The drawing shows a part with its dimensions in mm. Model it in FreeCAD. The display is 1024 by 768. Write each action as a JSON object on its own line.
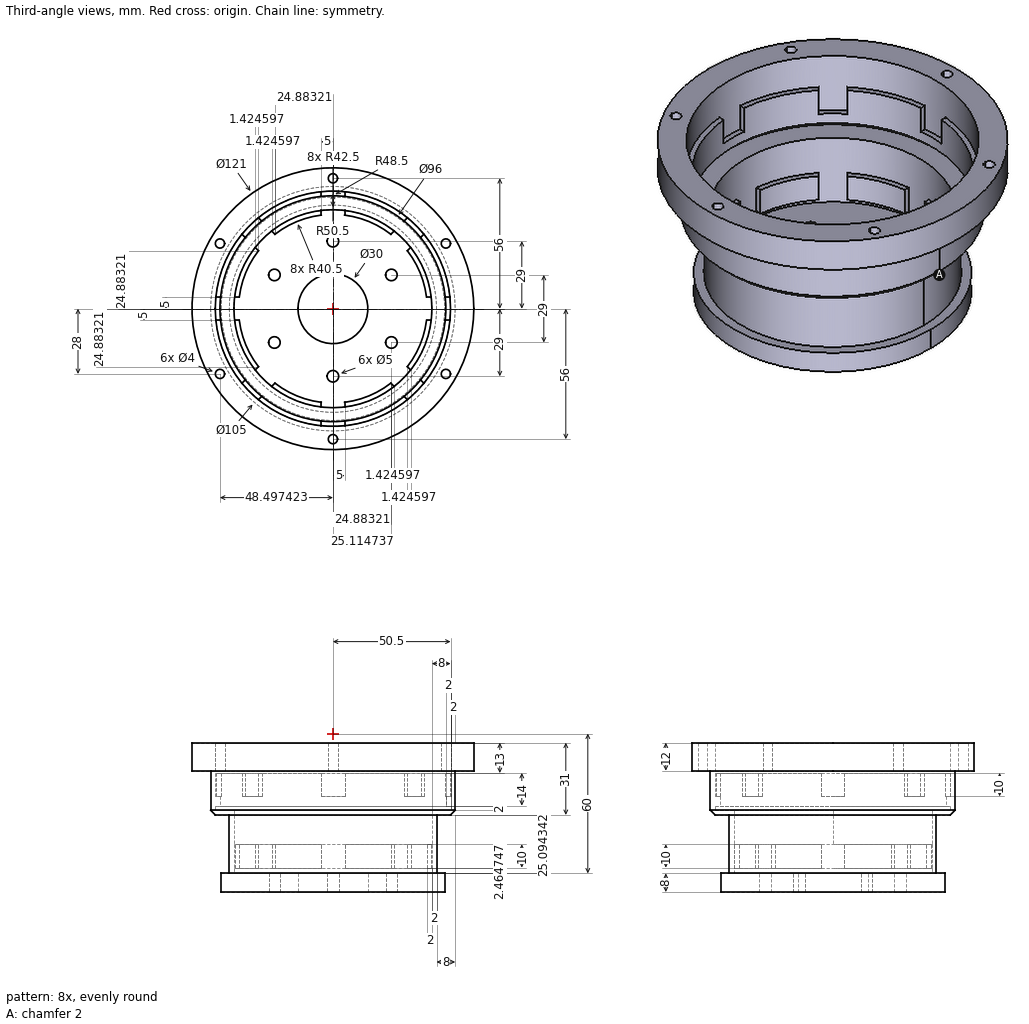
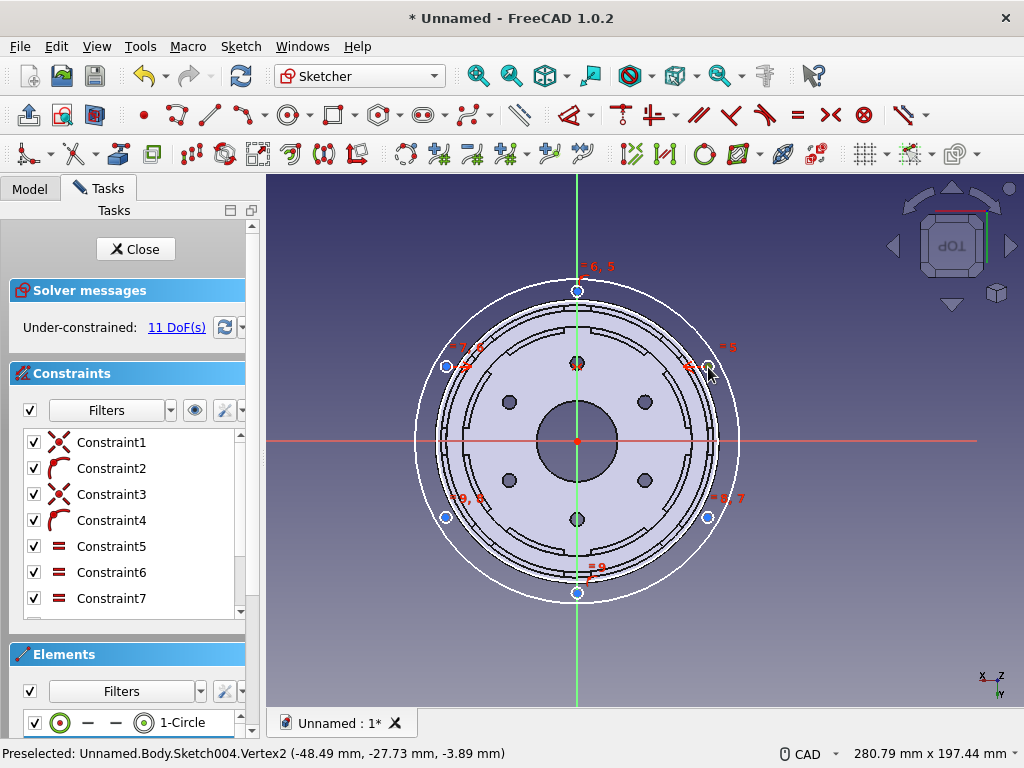
{"action": "left_click", "coordinate": [708, 518]}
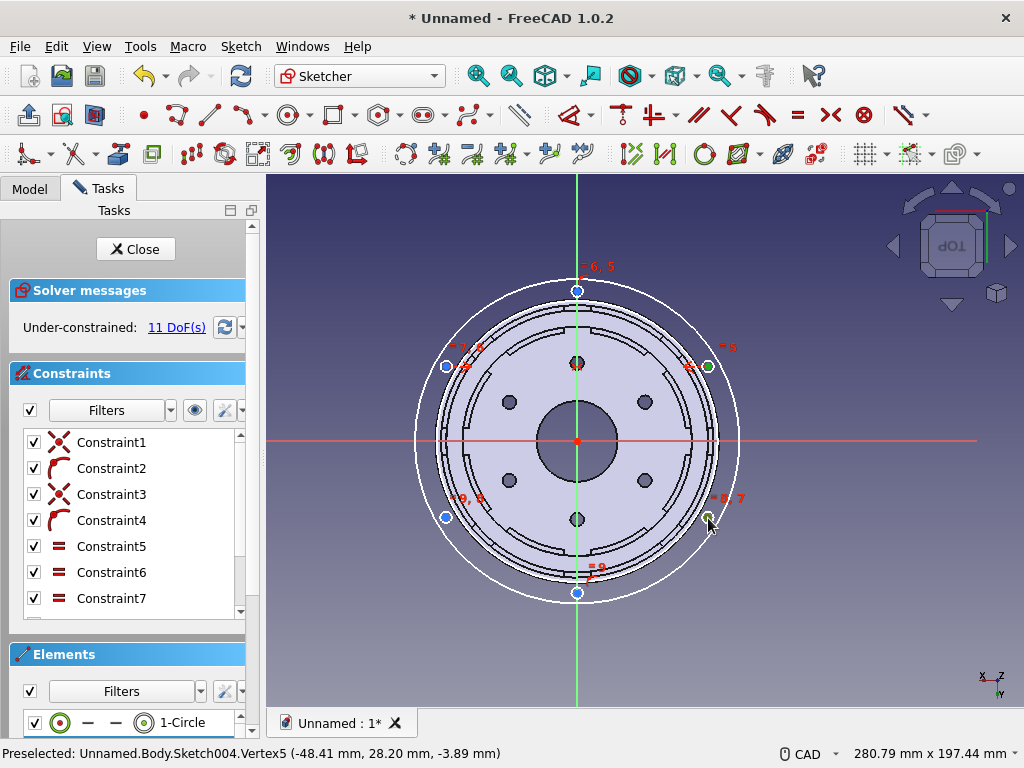
{"action": "left_click", "coordinate": [334, 441]}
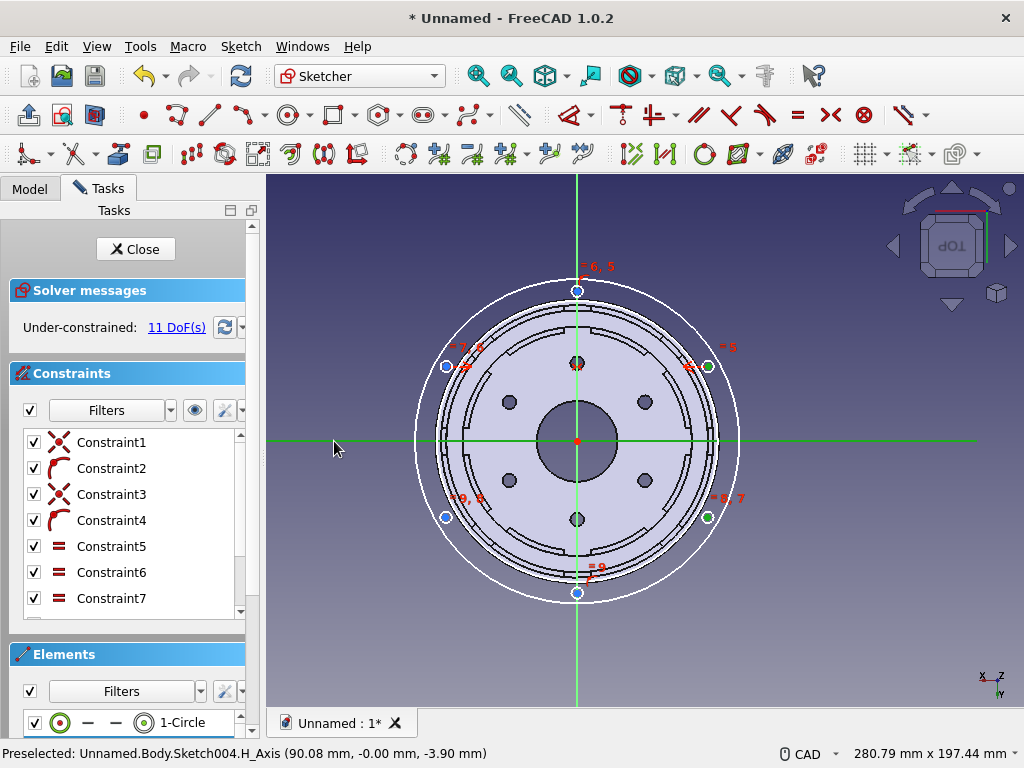
{"action": "key", "text": "s"}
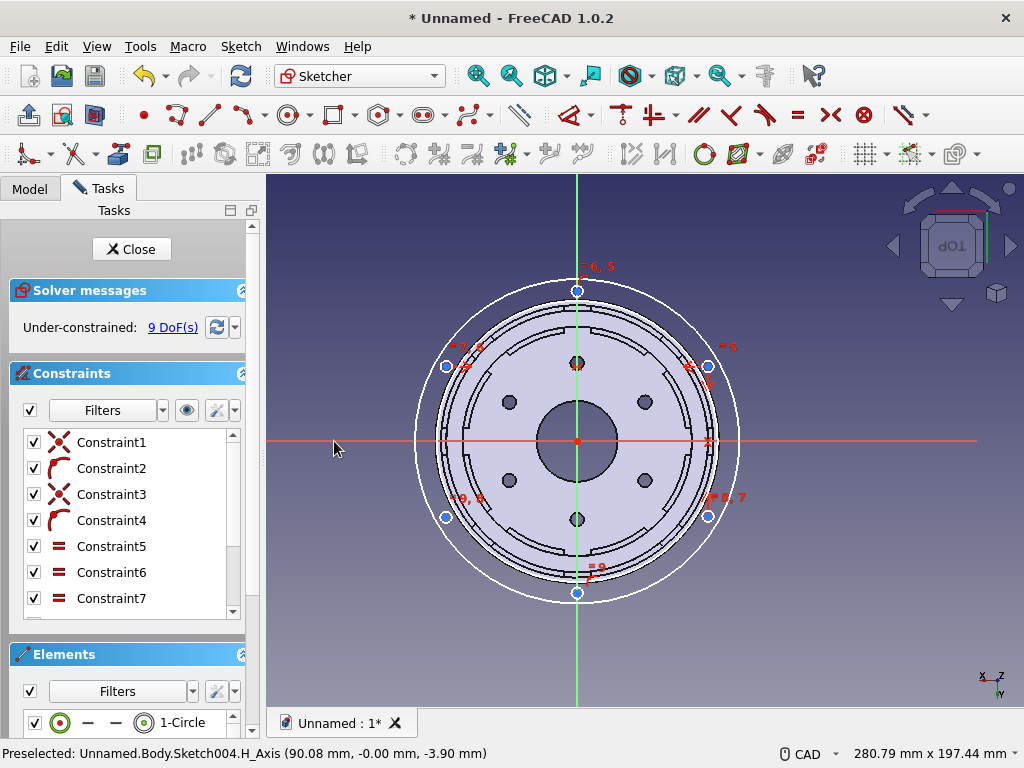
{"action": "left_click", "coordinate": [446, 367]}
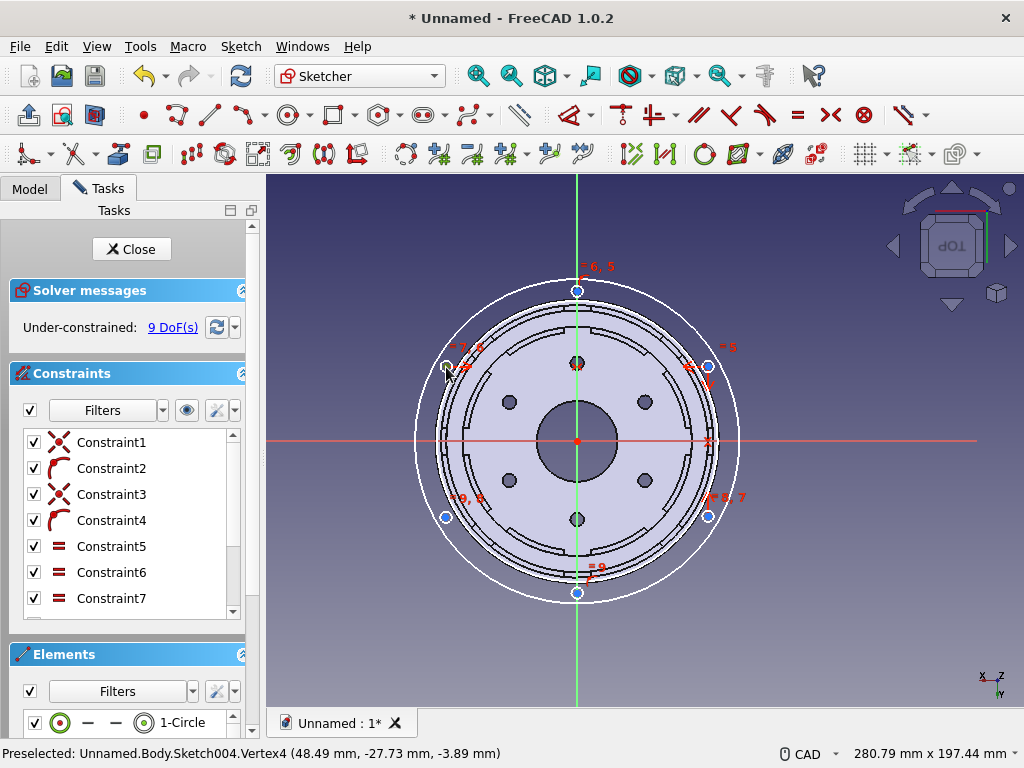
{"action": "left_click", "coordinate": [446, 517]}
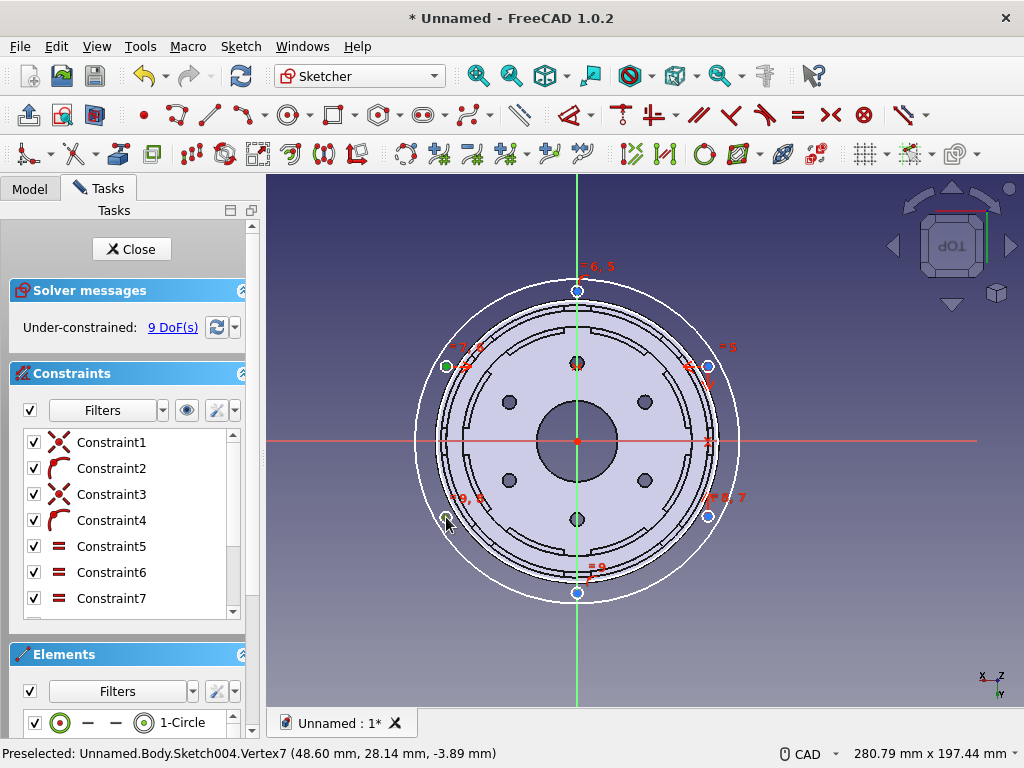
{"action": "left_click", "coordinate": [334, 441]}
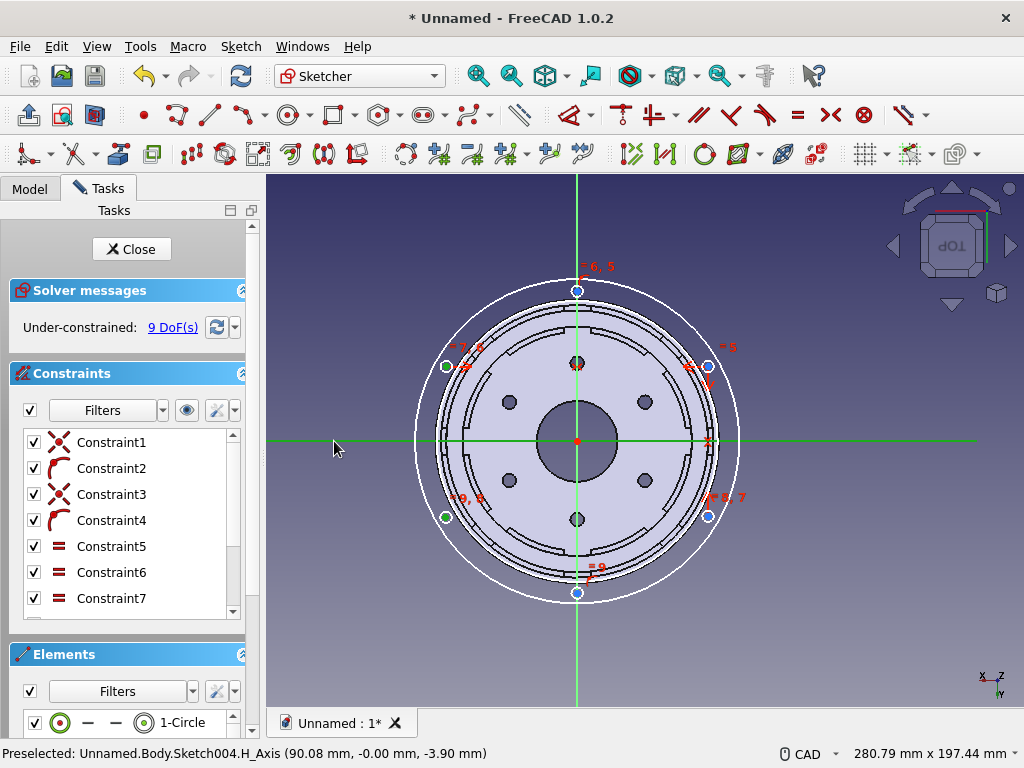
{"action": "key", "text": "s"}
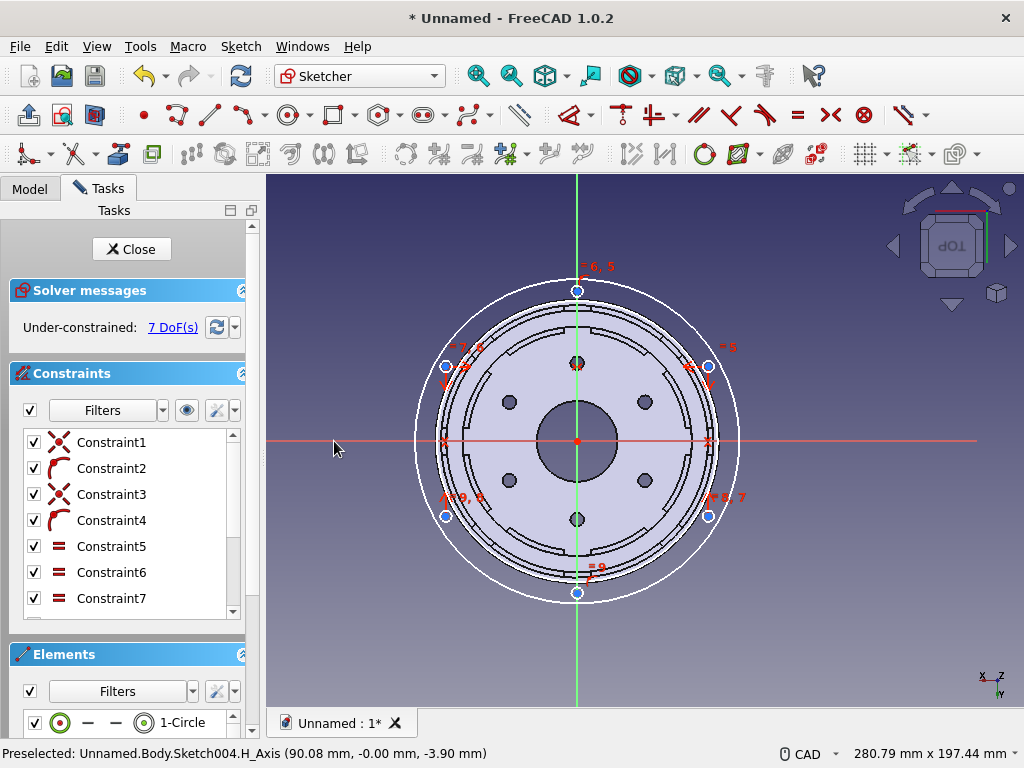
{"action": "key", "text": "d"}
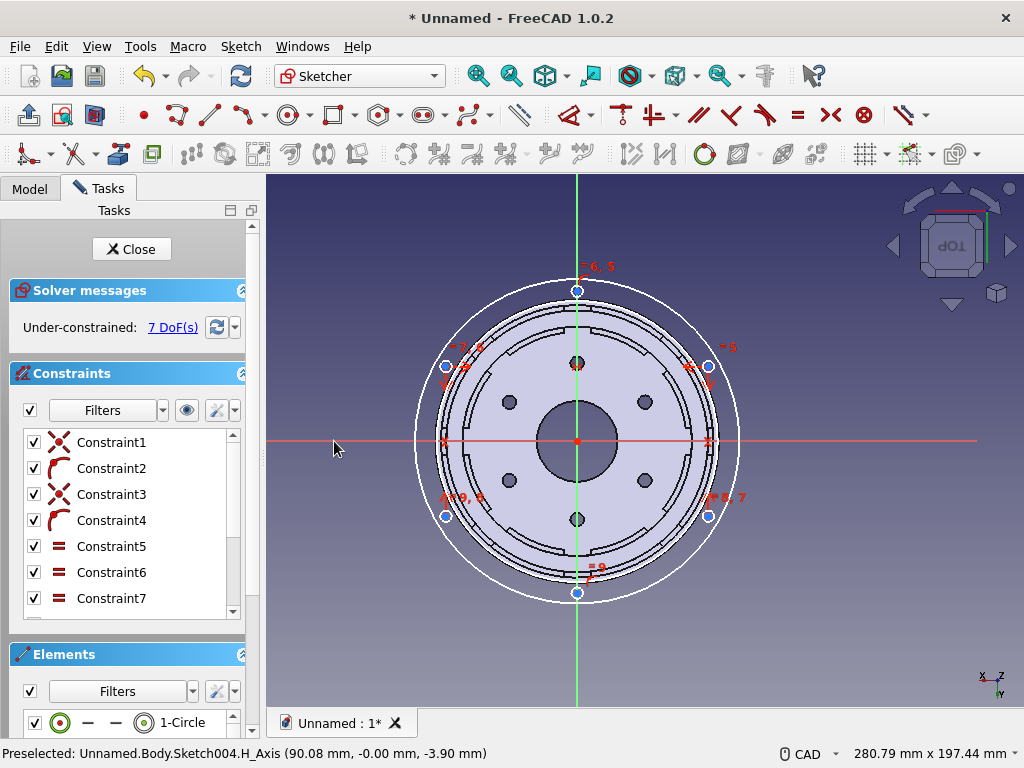
{"action": "left_click", "coordinate": [692, 326]}
{"action": "left_click", "coordinate": [715, 303]}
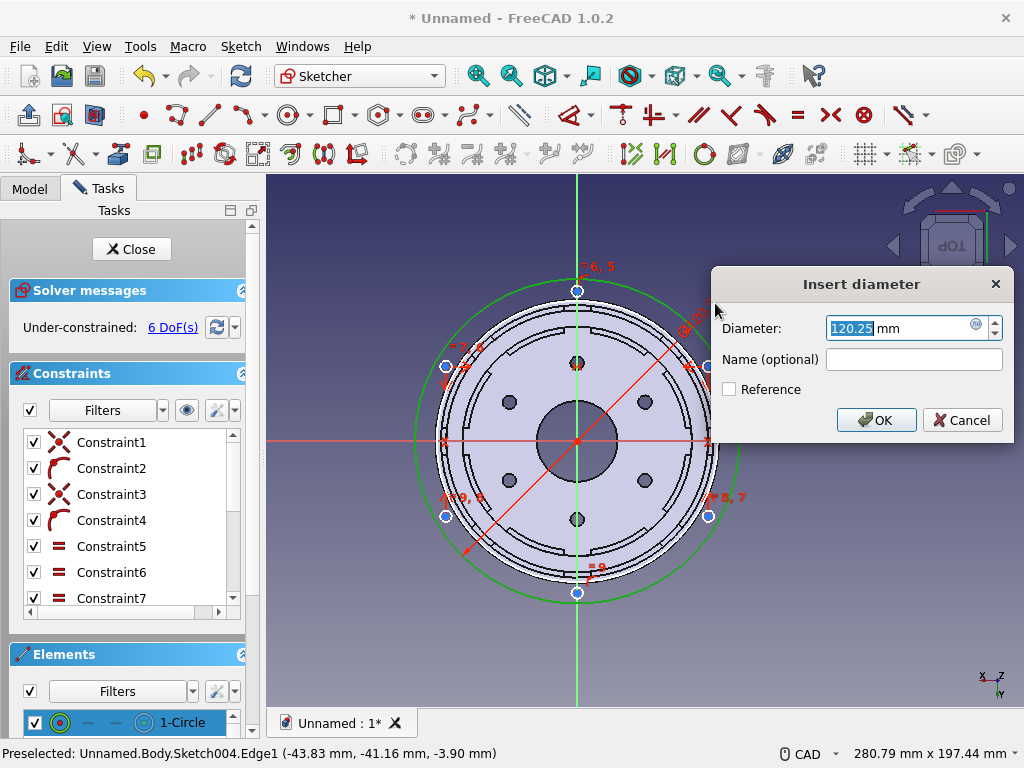
{"action": "type", "text": "121"}
{"action": "key", "text": "Return"}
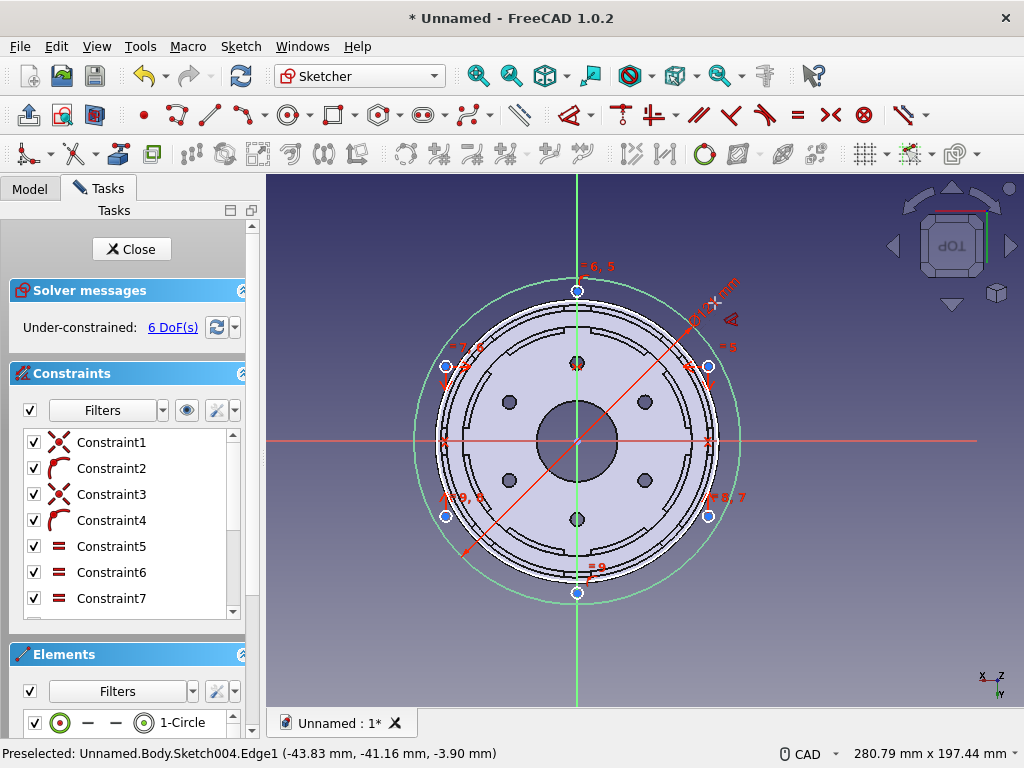
{"action": "scroll", "coordinate": [704, 363], "scroll_direction": "up", "scroll_amount": 7}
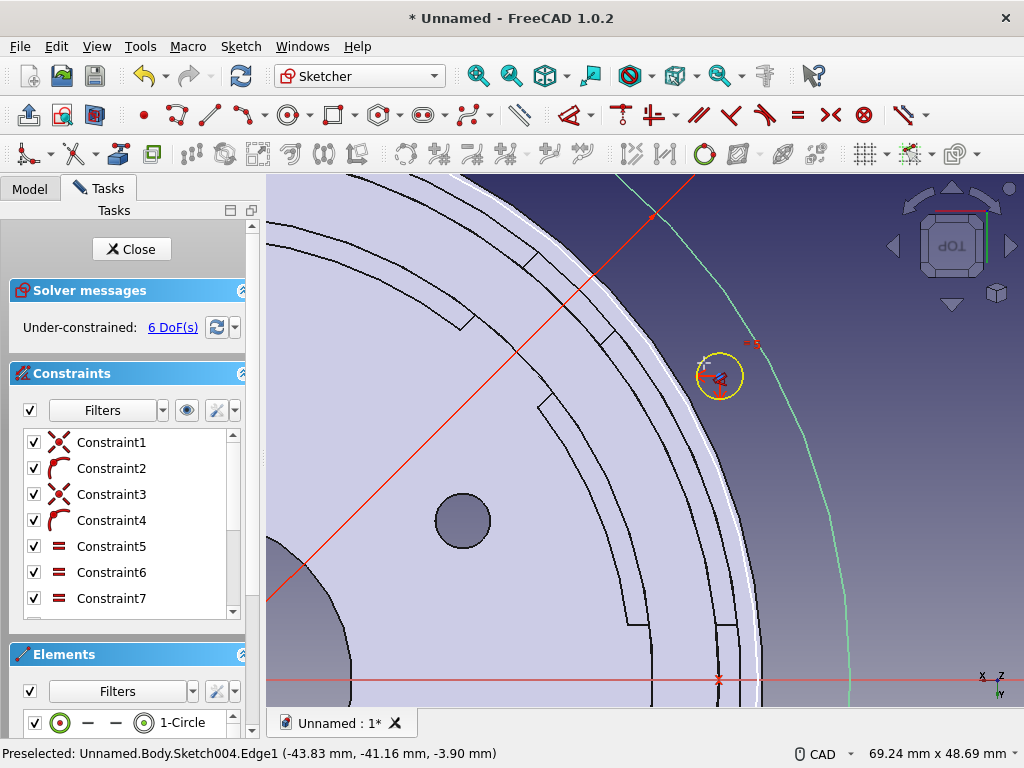
{"action": "left_click", "coordinate": [704, 360]}
{"action": "left_click", "coordinate": [682, 337]}